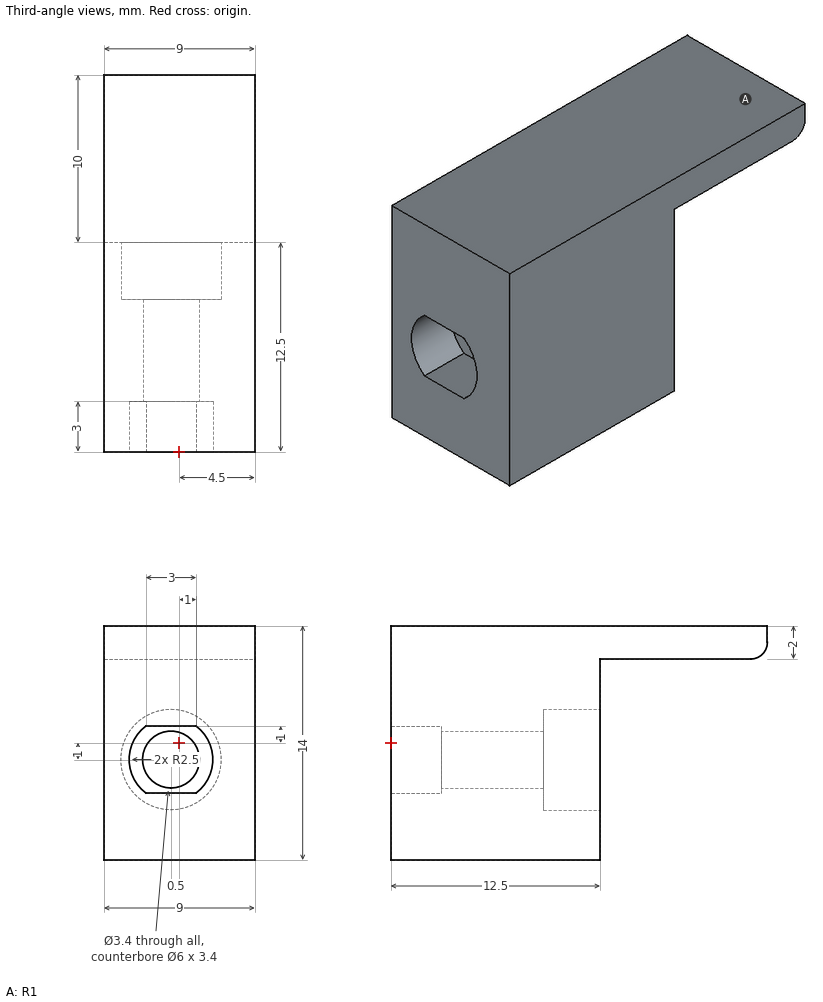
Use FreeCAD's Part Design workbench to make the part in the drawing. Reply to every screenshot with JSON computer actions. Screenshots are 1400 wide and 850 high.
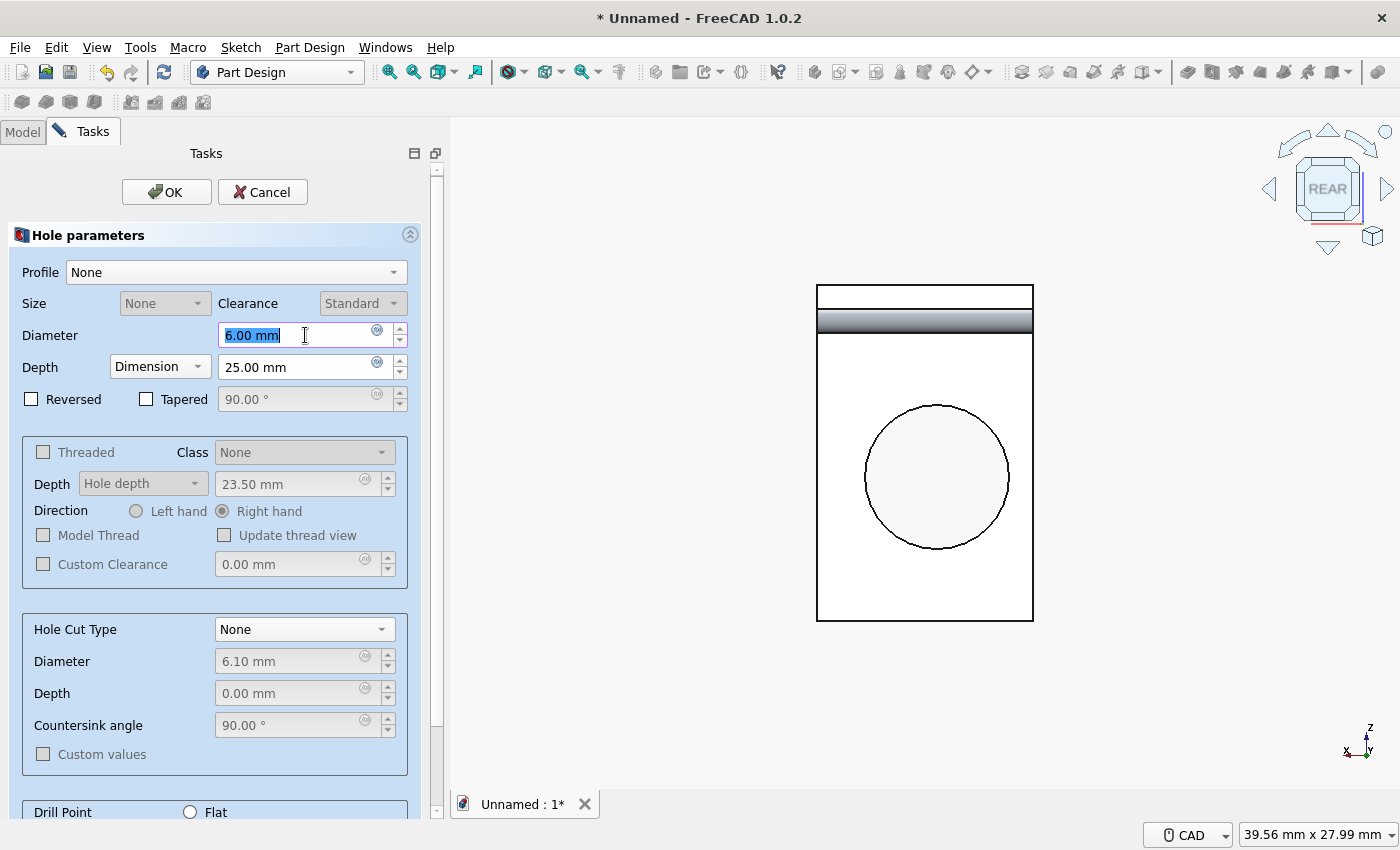
{"action": "type", "text": "3.4"}
{"action": "key", "text": "Tab"}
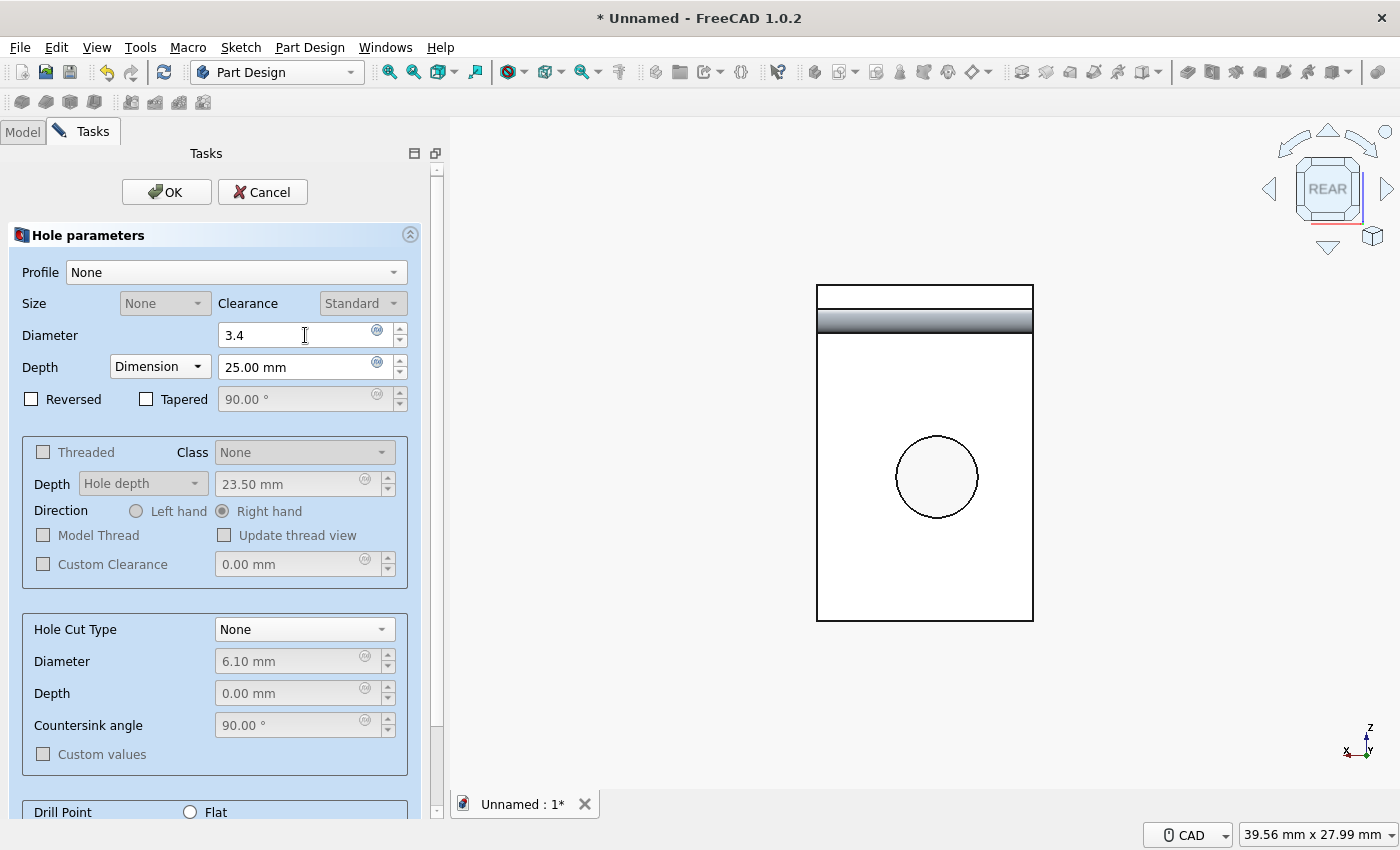
{"action": "left_click", "coordinate": [161, 366]}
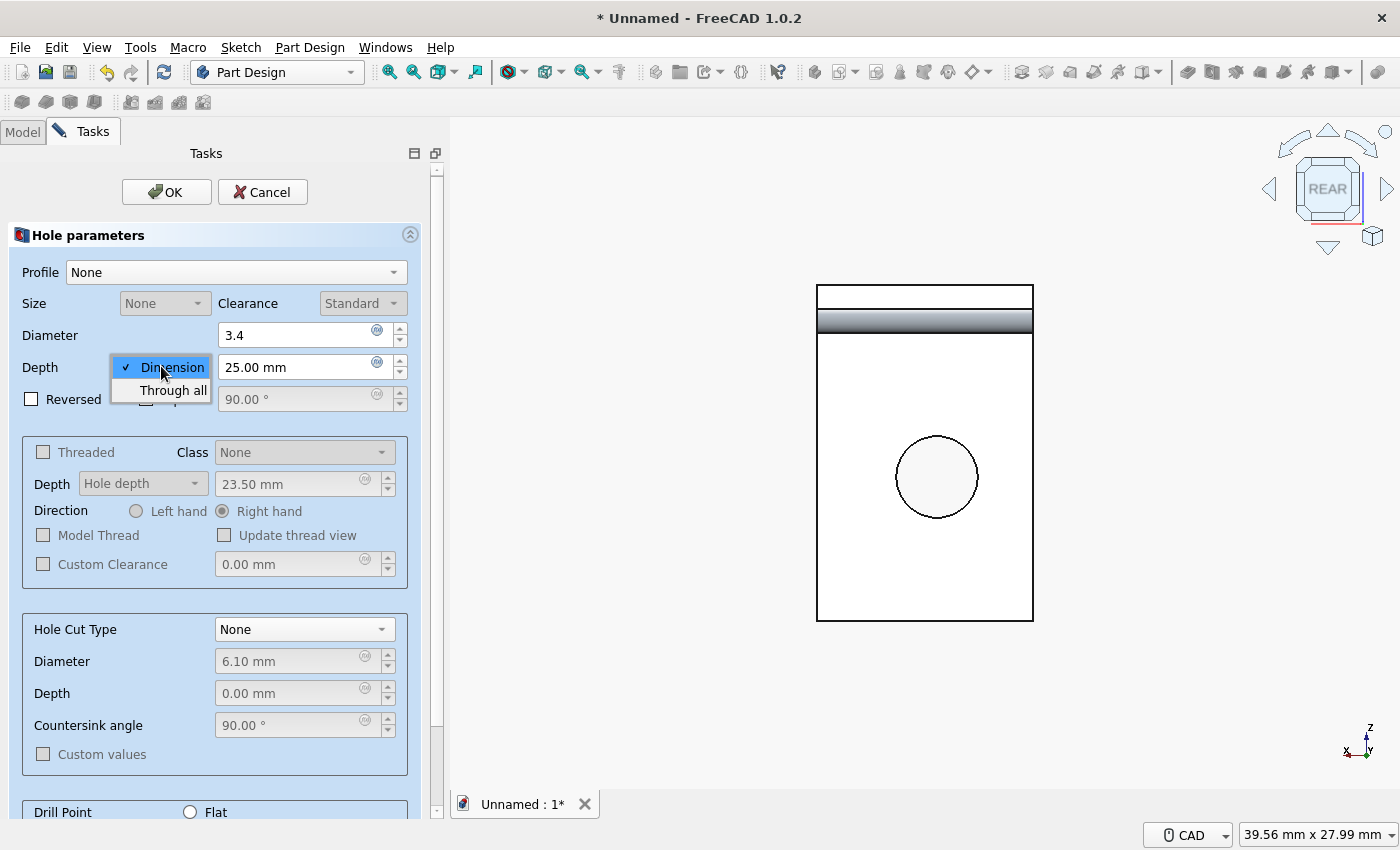
{"action": "left_click", "coordinate": [160, 390]}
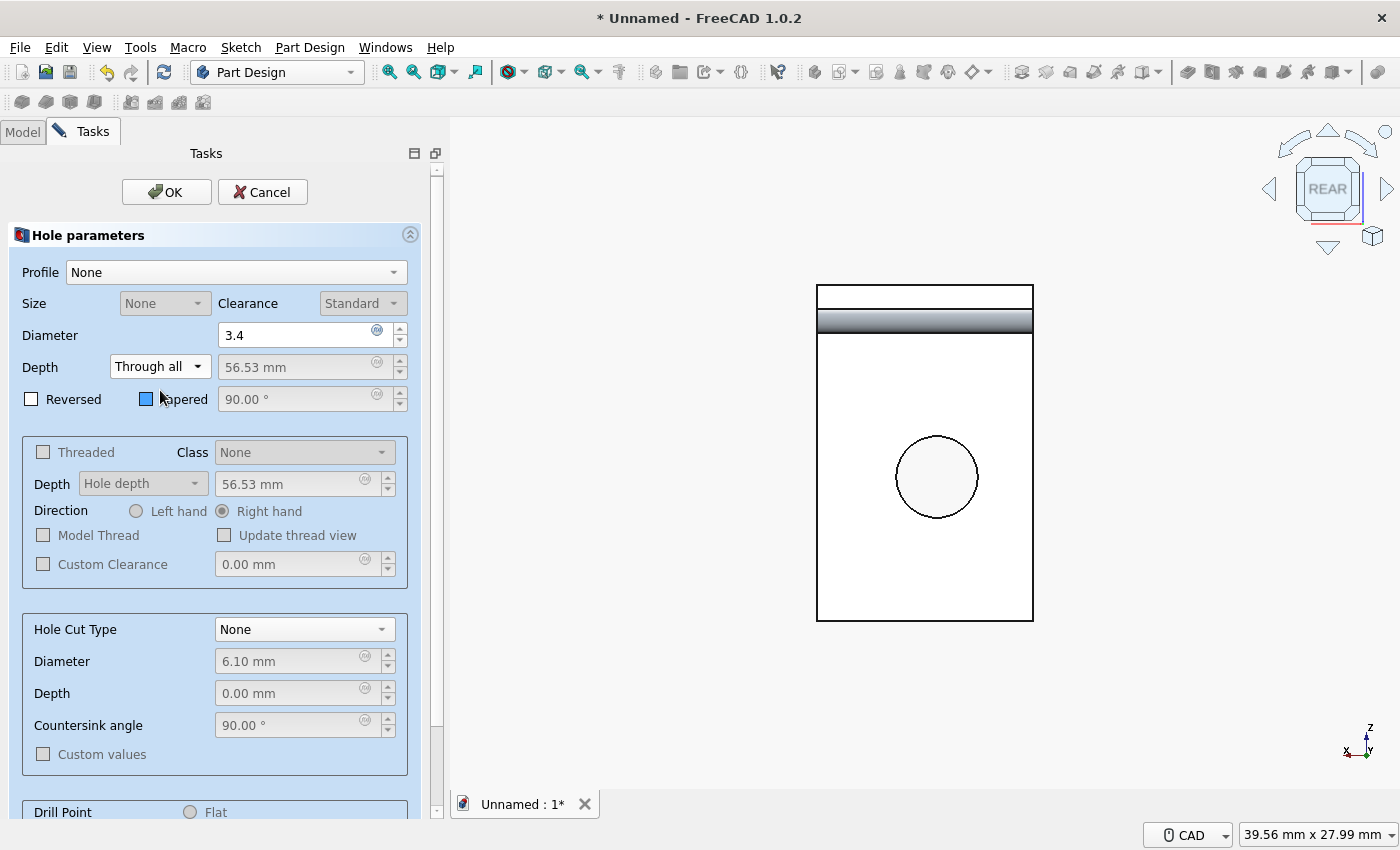
{"action": "left_click", "coordinate": [306, 630]}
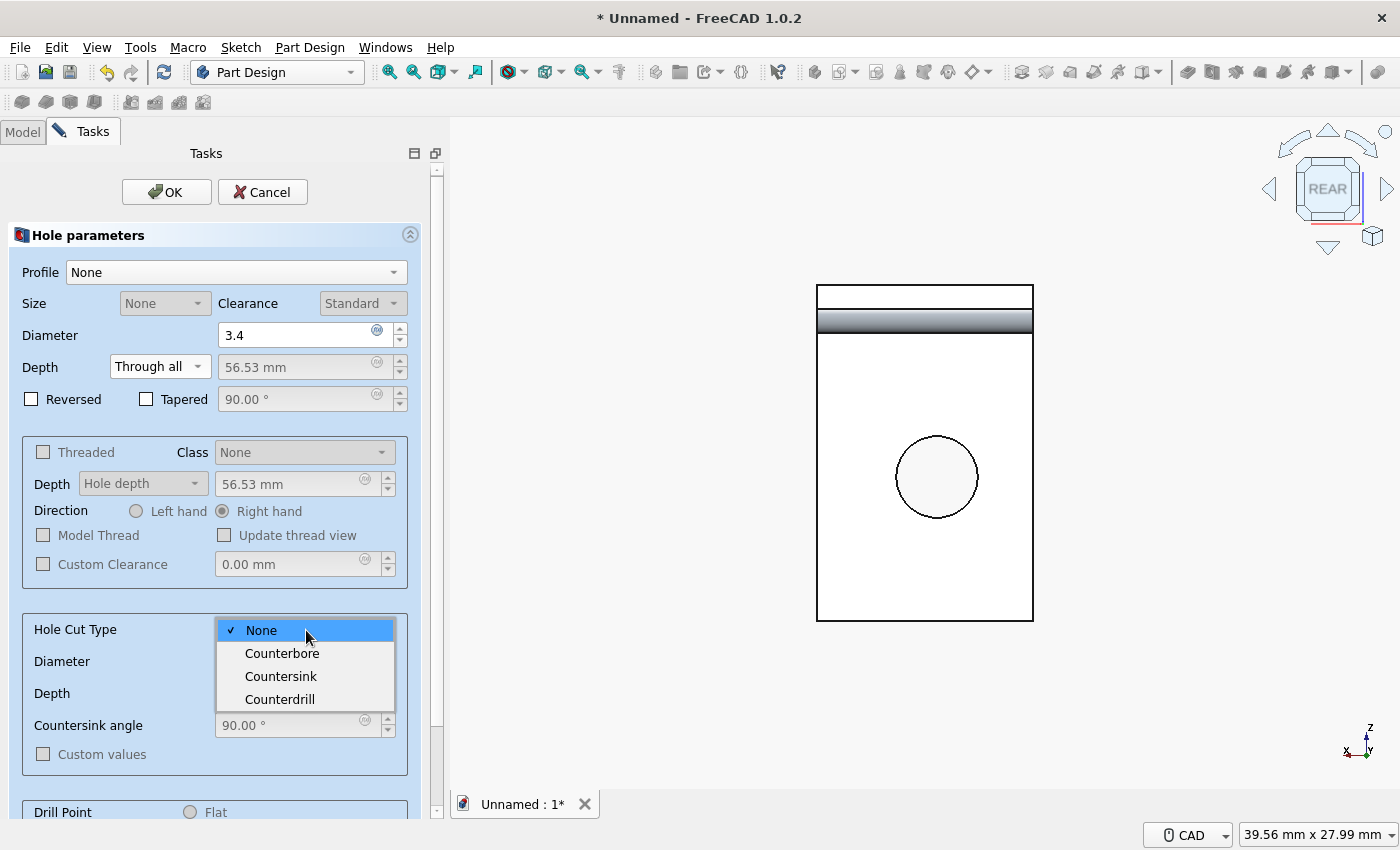
{"action": "left_click", "coordinate": [304, 654]}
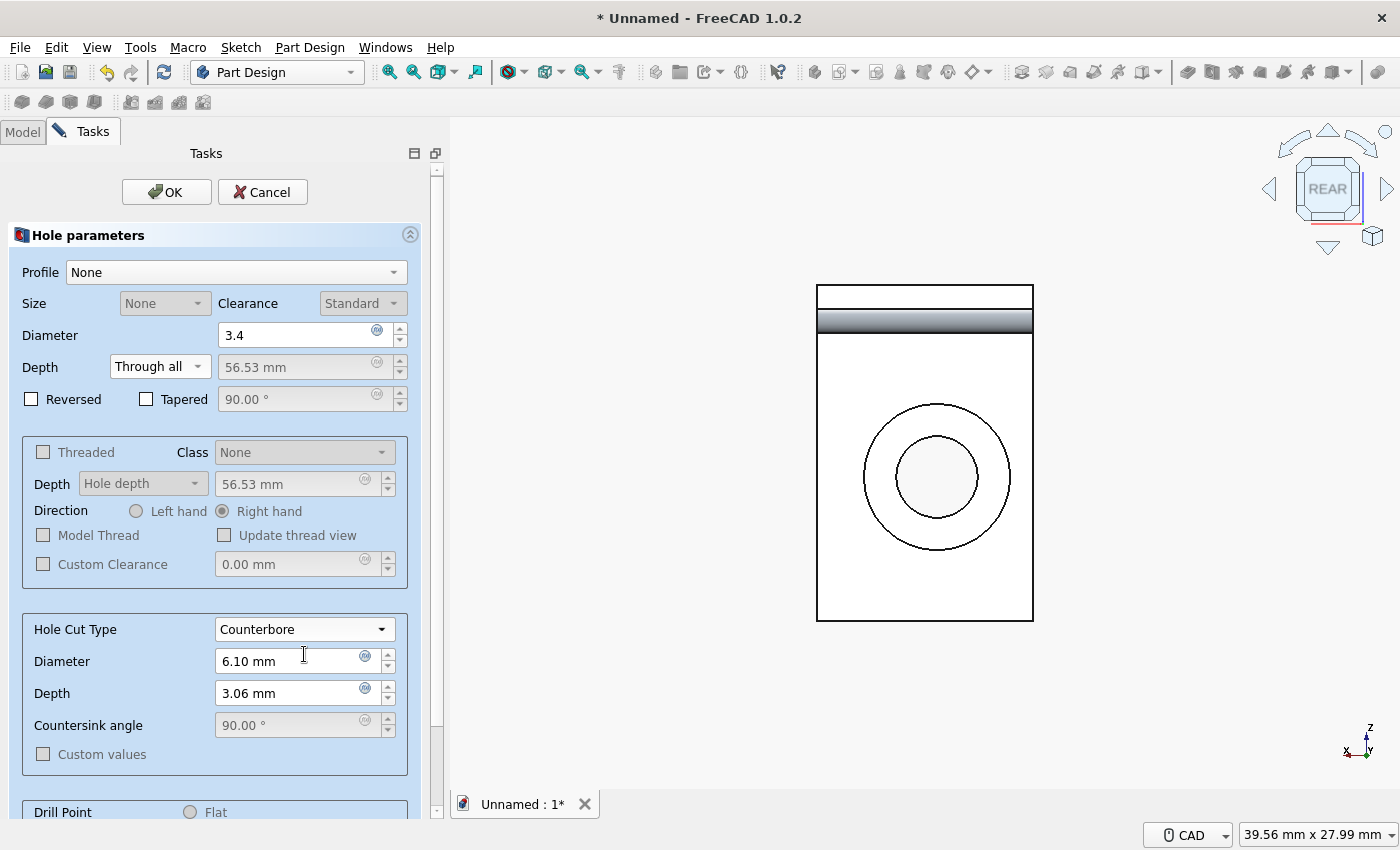
{"action": "triple_click", "coordinate": [298, 661]}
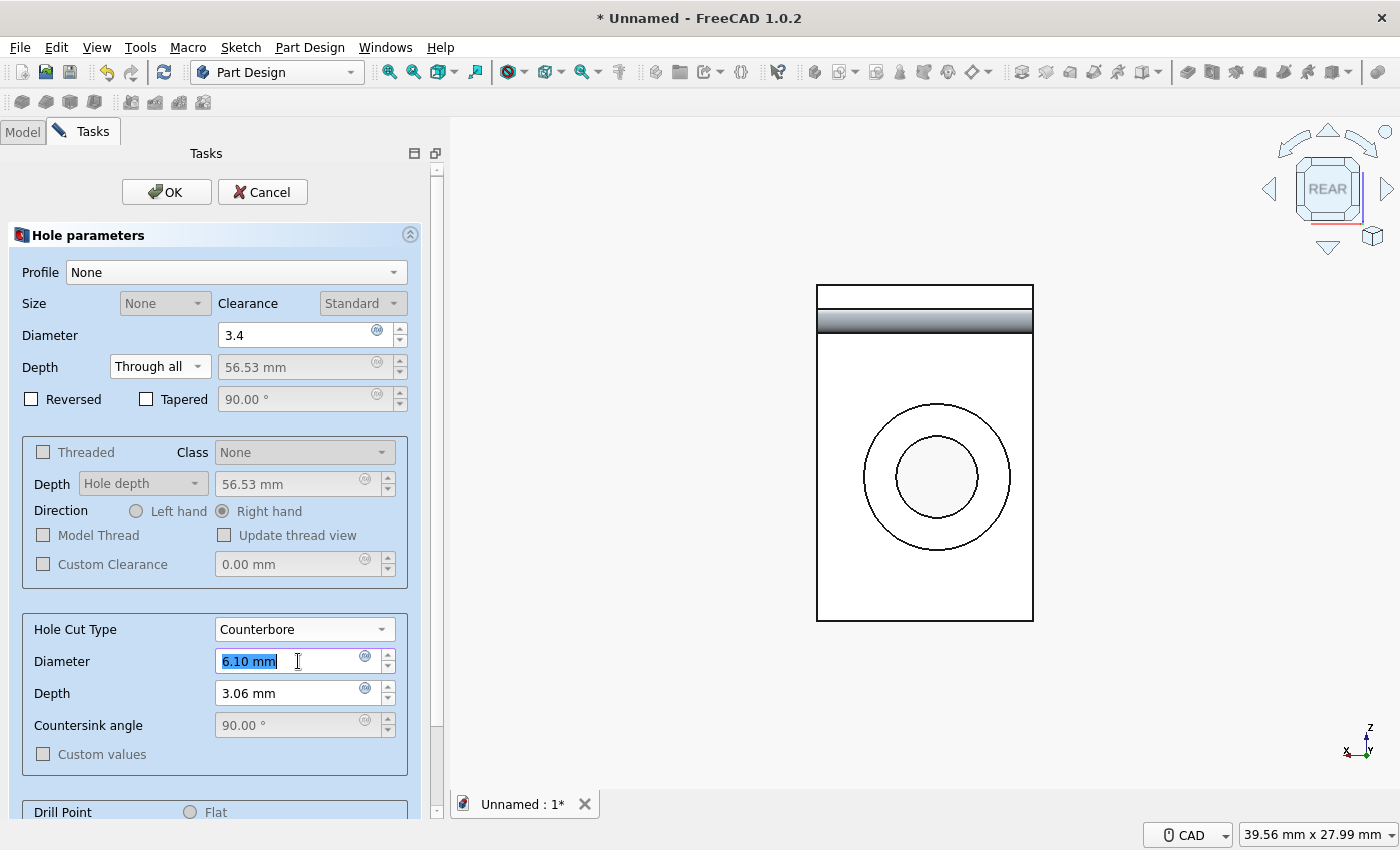
{"action": "type", "text": "6"}
{"action": "key", "text": "Tab"}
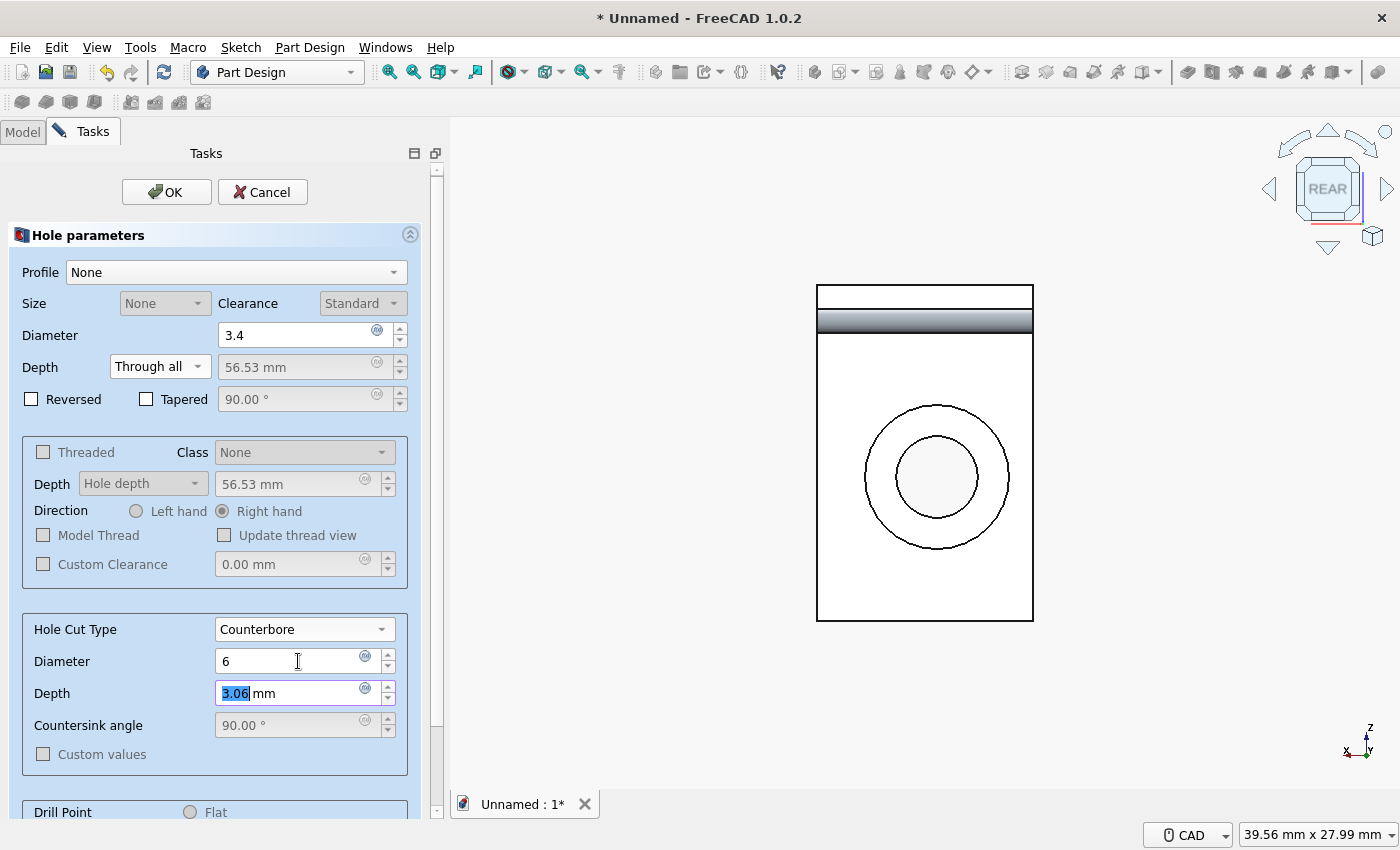
{"action": "type", "text": "3.4"}
{"action": "key", "text": "Tab"}